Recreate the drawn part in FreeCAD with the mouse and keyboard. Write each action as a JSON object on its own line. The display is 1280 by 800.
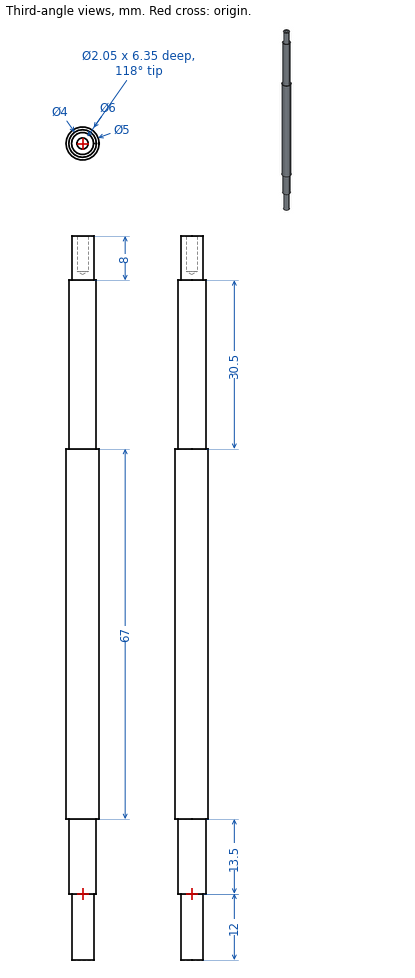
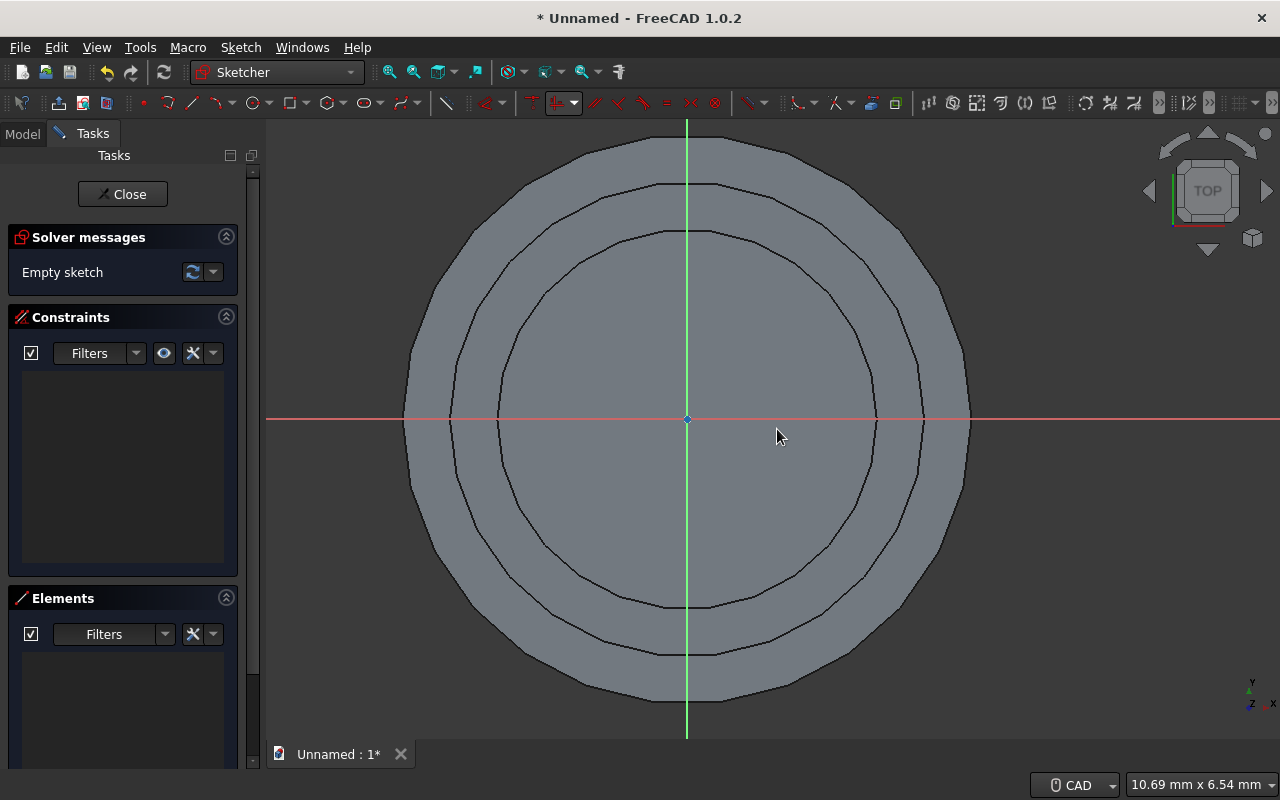
{"action": "scroll", "coordinate": [673, 412], "scroll_direction": "up", "scroll_amount": 4}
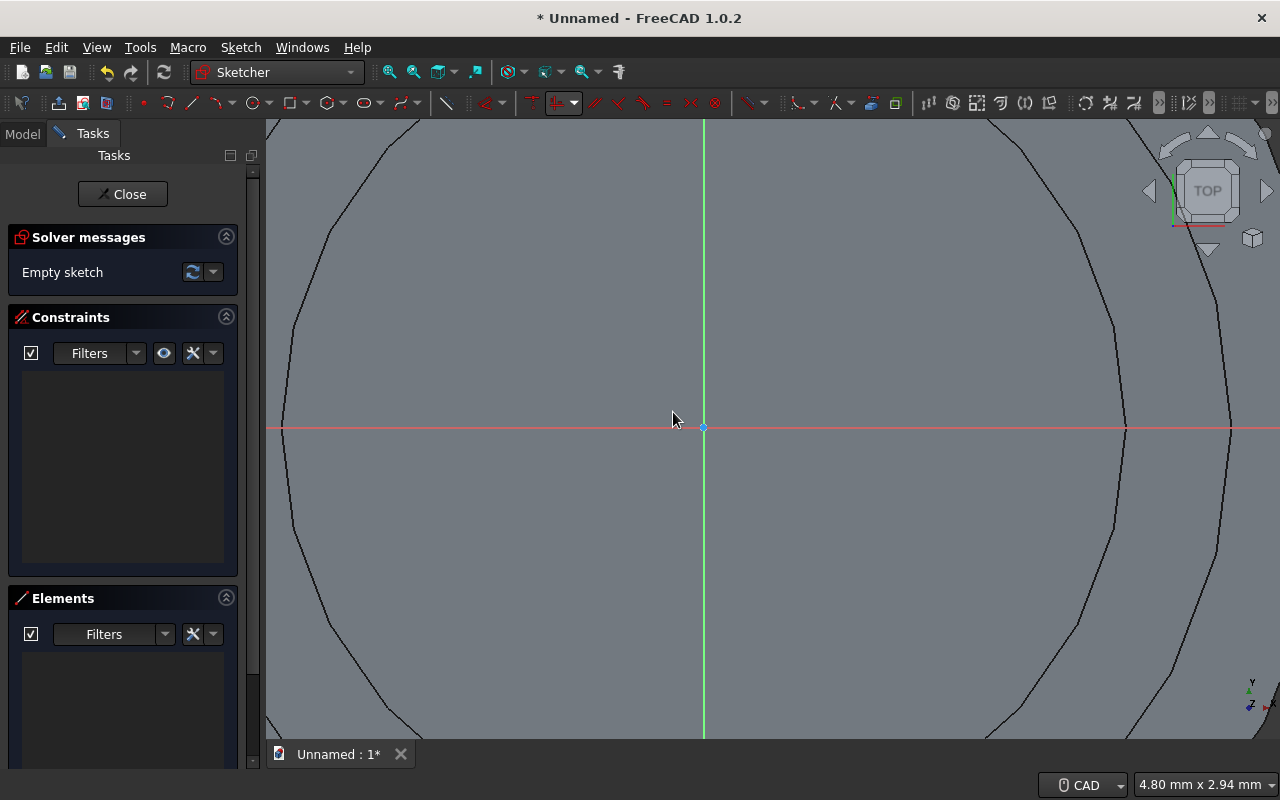
{"action": "key", "text": "g c"}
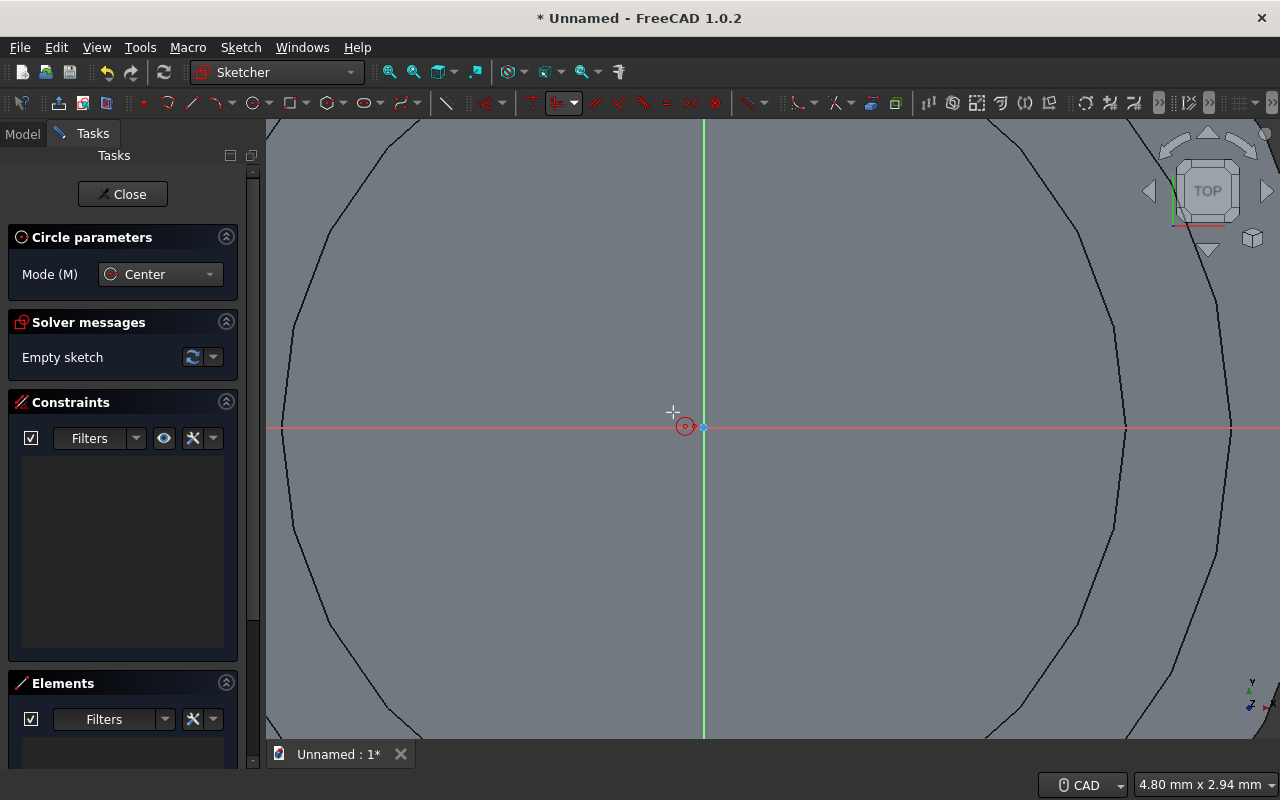
{"action": "left_click", "coordinate": [704, 428]}
{"action": "left_click", "coordinate": [857, 275]}
{"action": "key", "text": "Escape"}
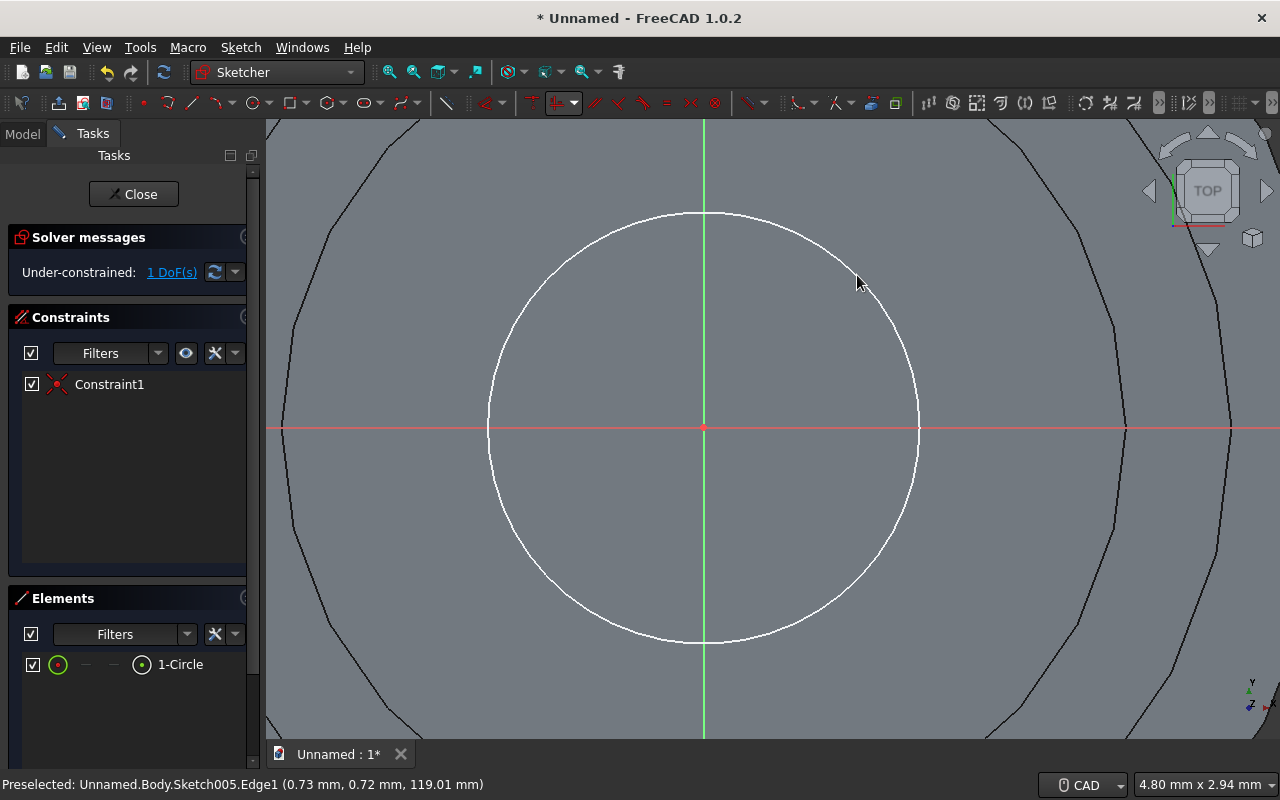
{"action": "left_click", "coordinate": [486, 104]}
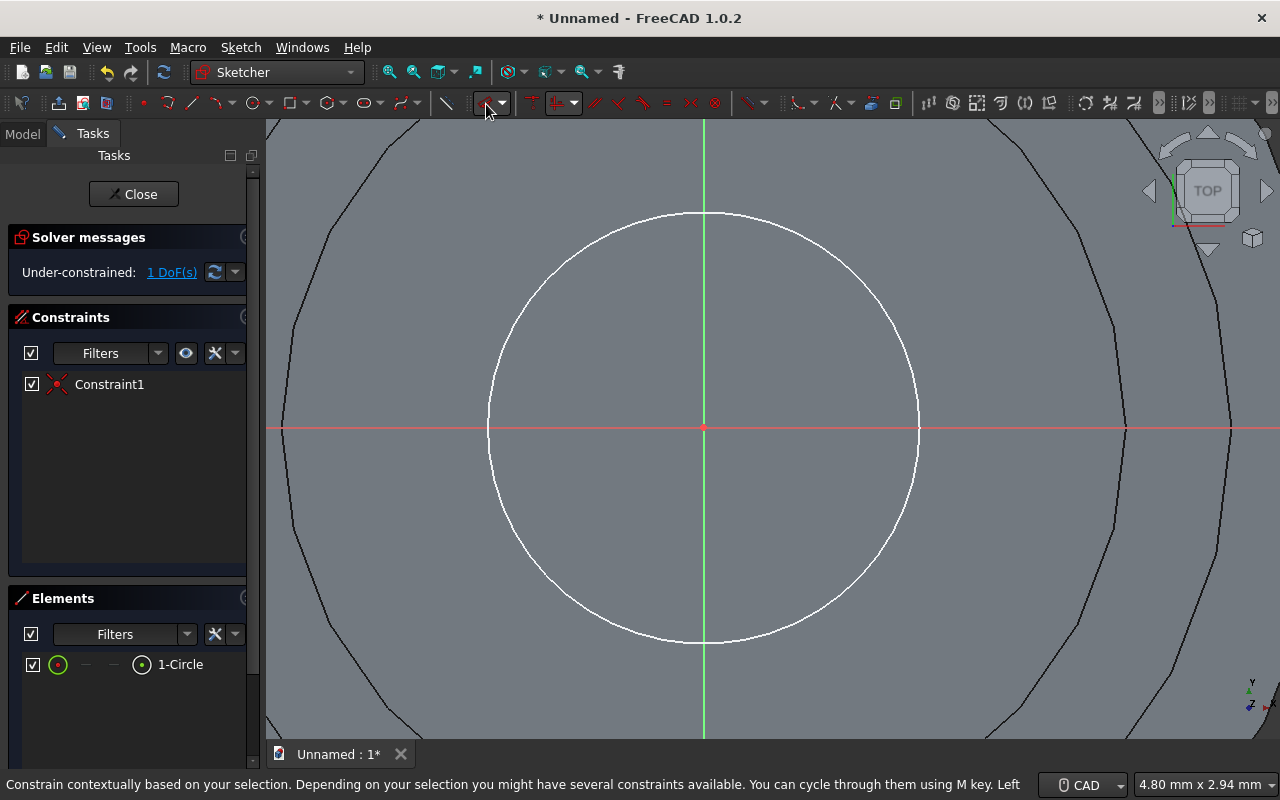
{"action": "left_click", "coordinate": [856, 275]}
{"action": "left_click", "coordinate": [879, 252]}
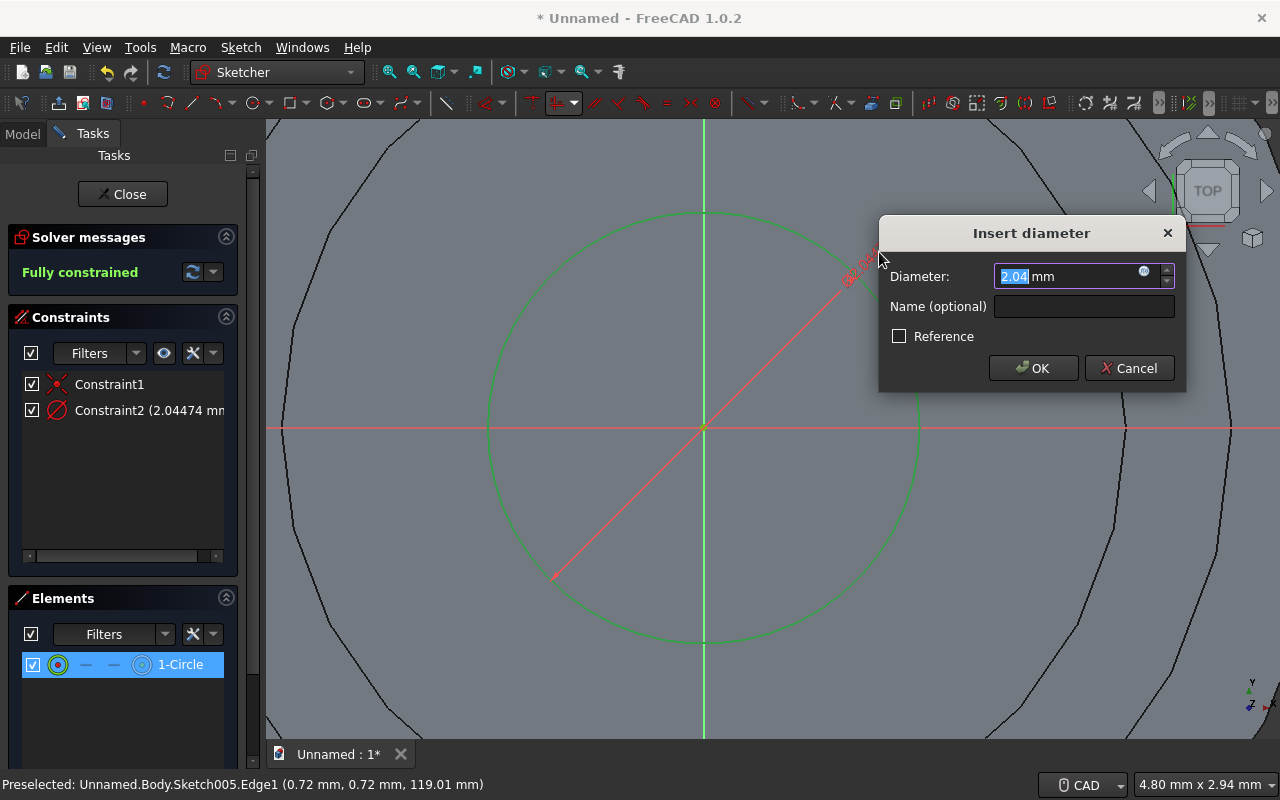
{"action": "type", "text": "2.05"}
{"action": "key", "text": "Return"}
{"action": "key", "text": "Escape"}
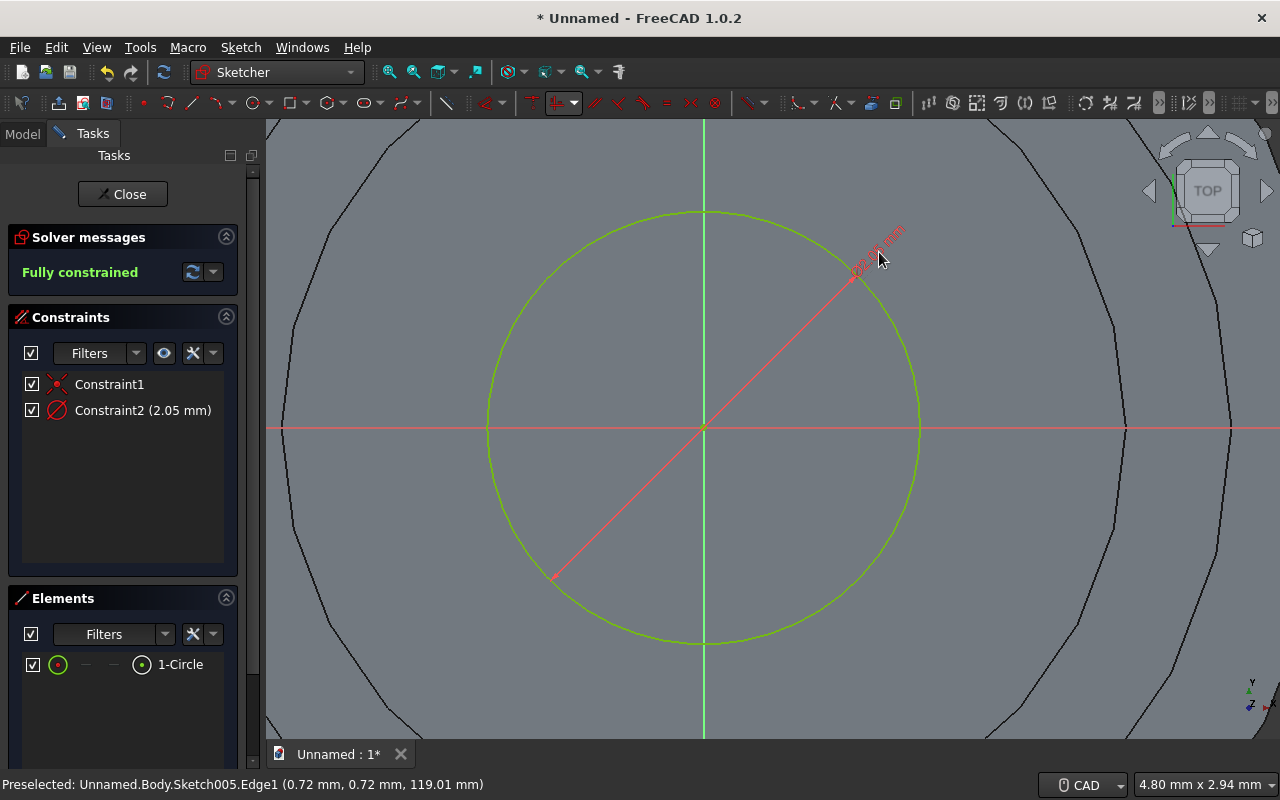
{"action": "left_click", "coordinate": [123, 194]}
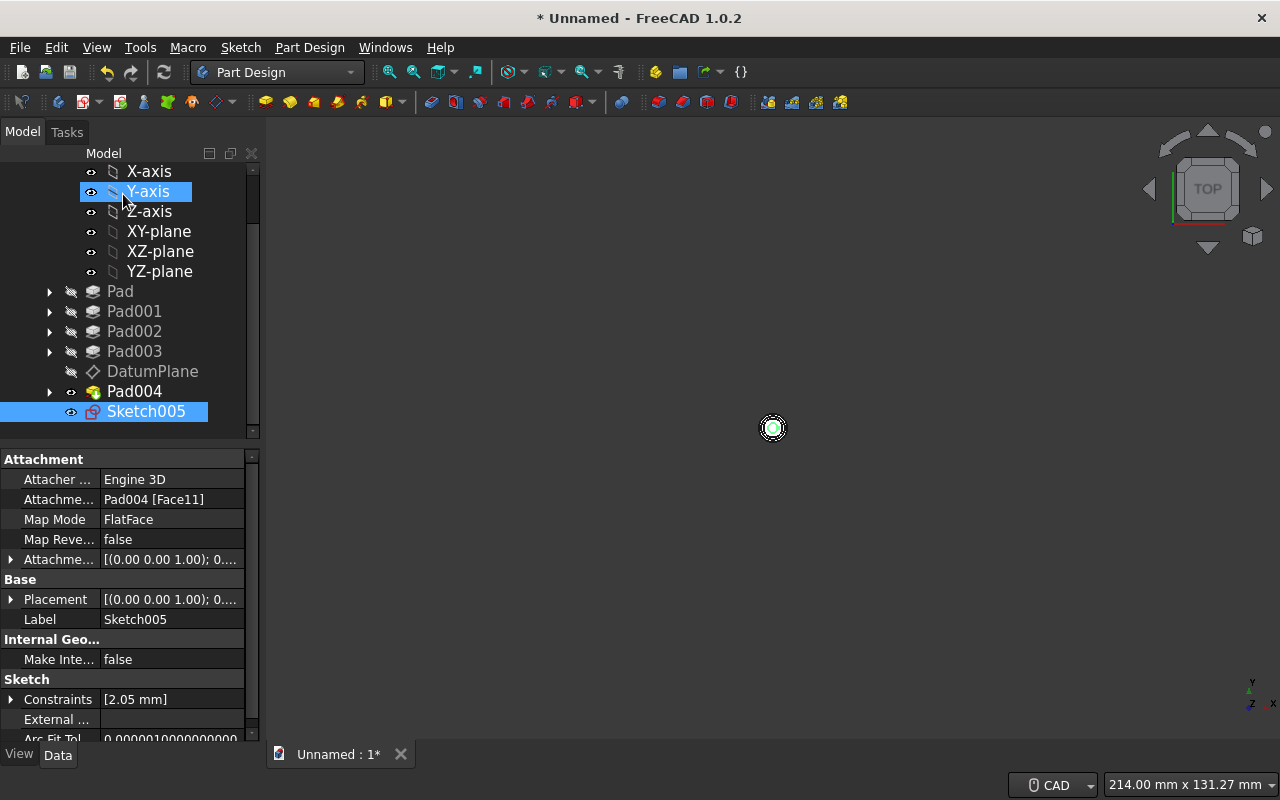
{"action": "left_click", "coordinate": [456, 102]}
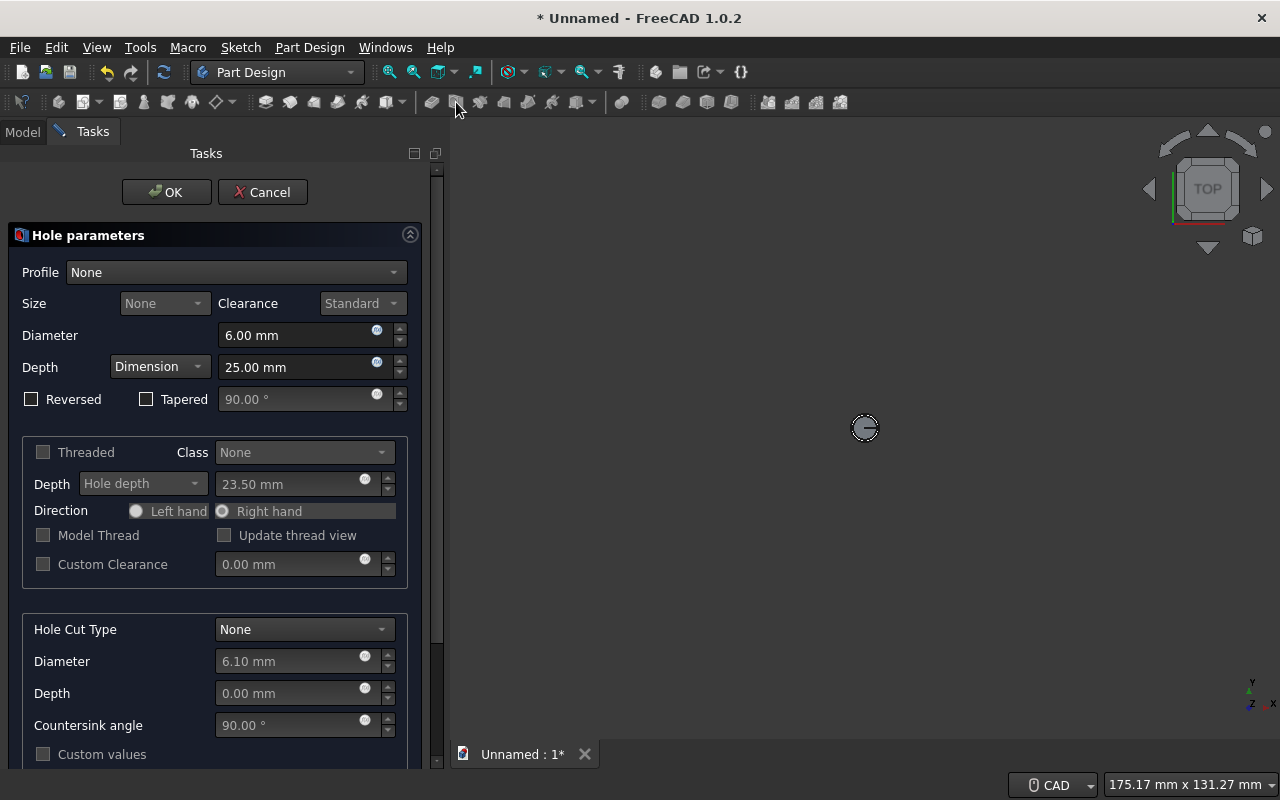
{"action": "triple_click", "coordinate": [305, 335]}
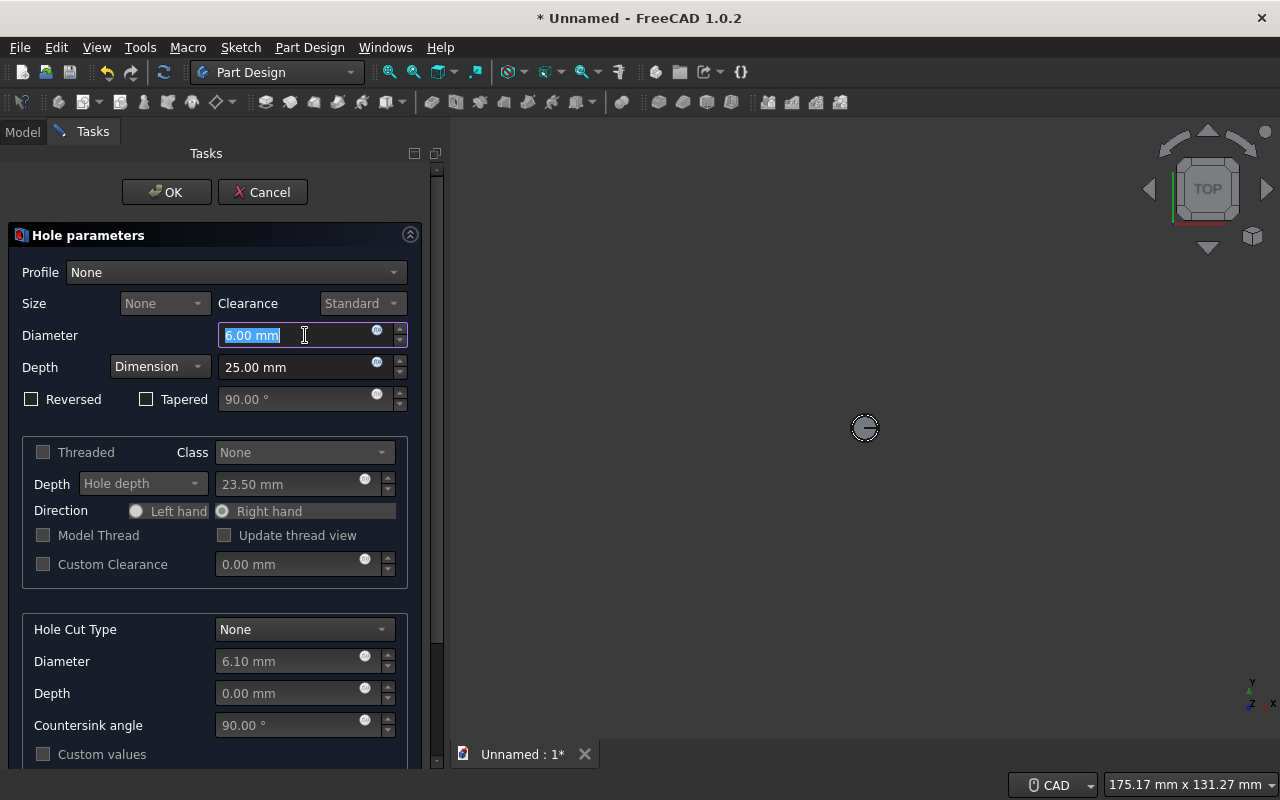
{"action": "type", "text": "2.05"}
{"action": "key", "text": "Tab"}